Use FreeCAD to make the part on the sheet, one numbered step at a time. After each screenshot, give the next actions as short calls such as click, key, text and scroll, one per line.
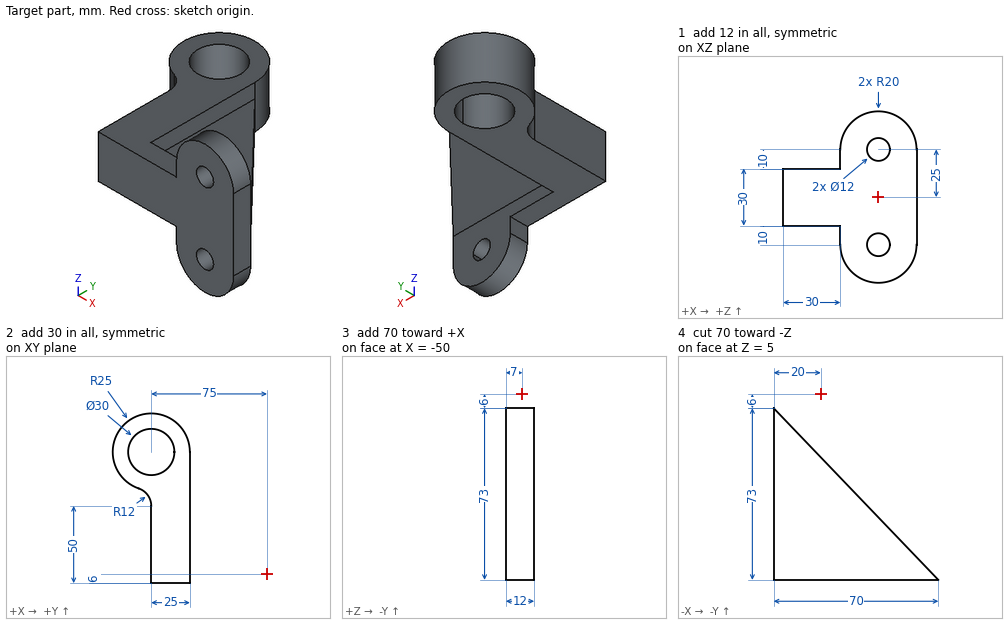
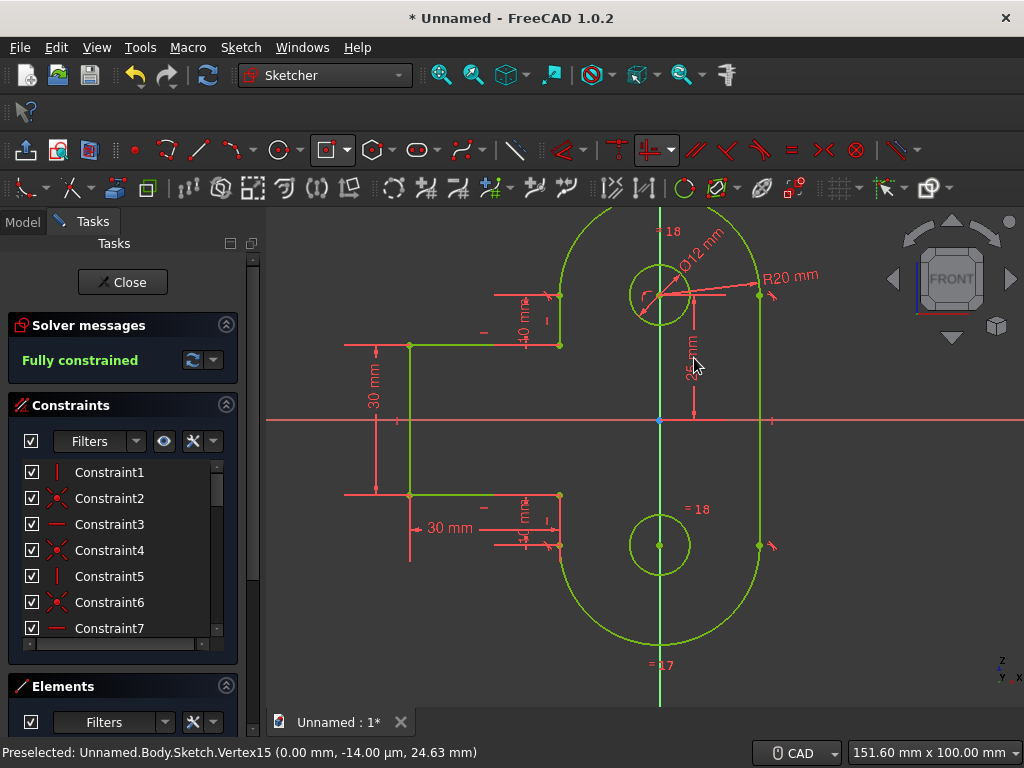
click(123, 282)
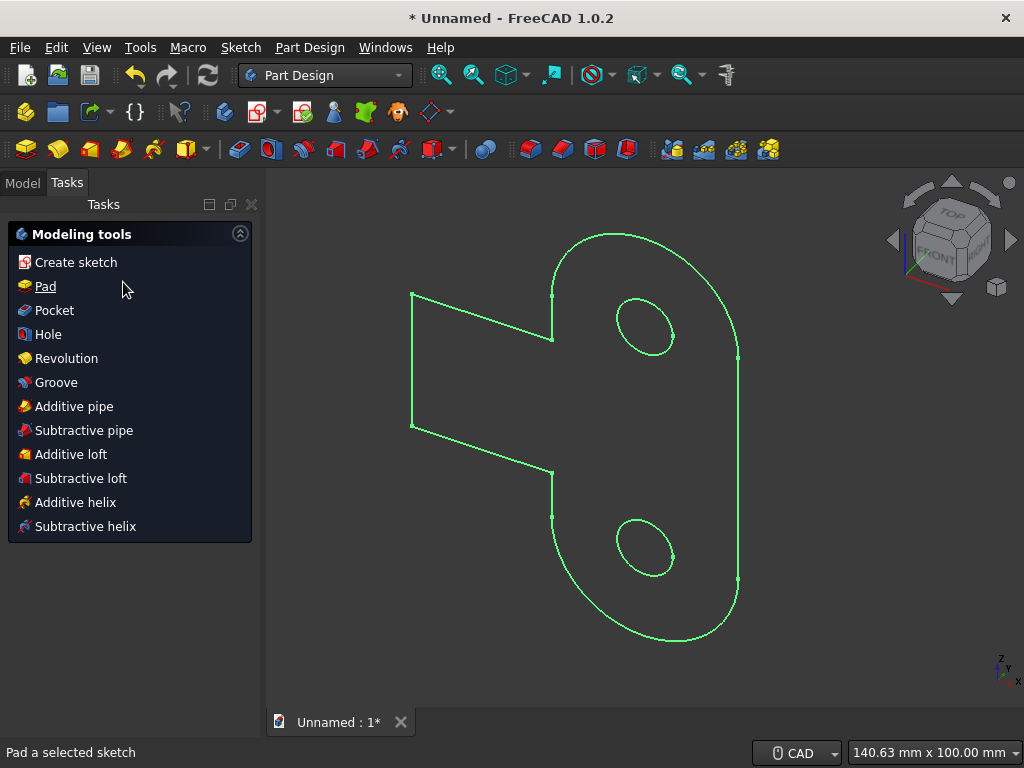
click(26, 150)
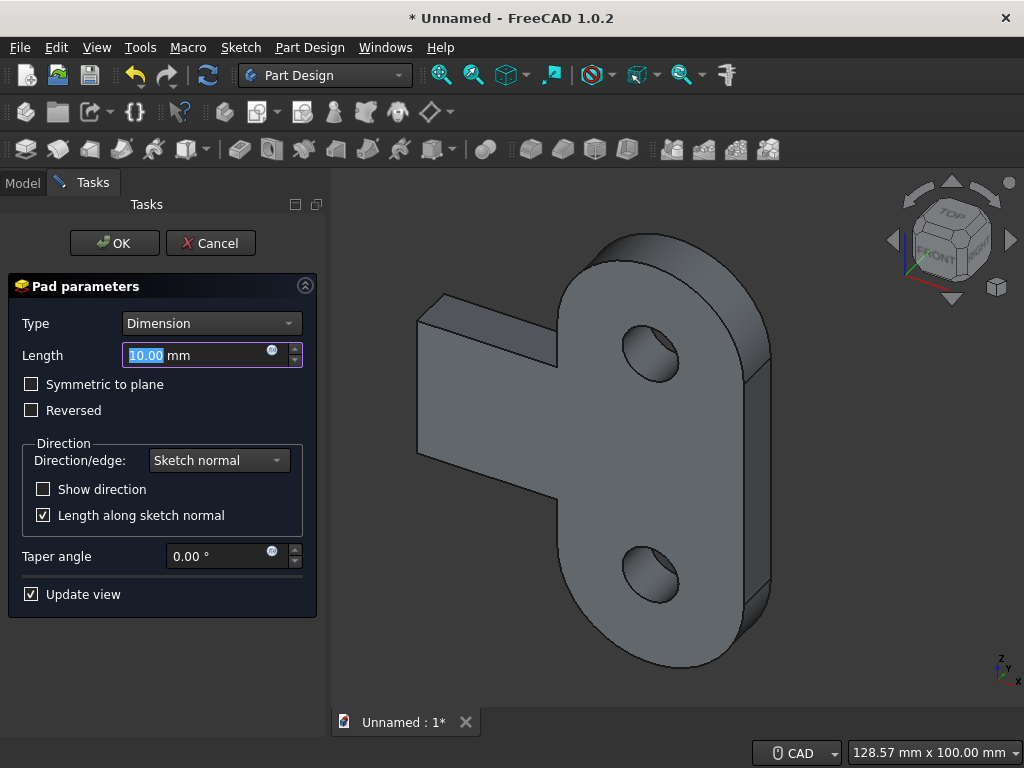
text(12)
key(Tab)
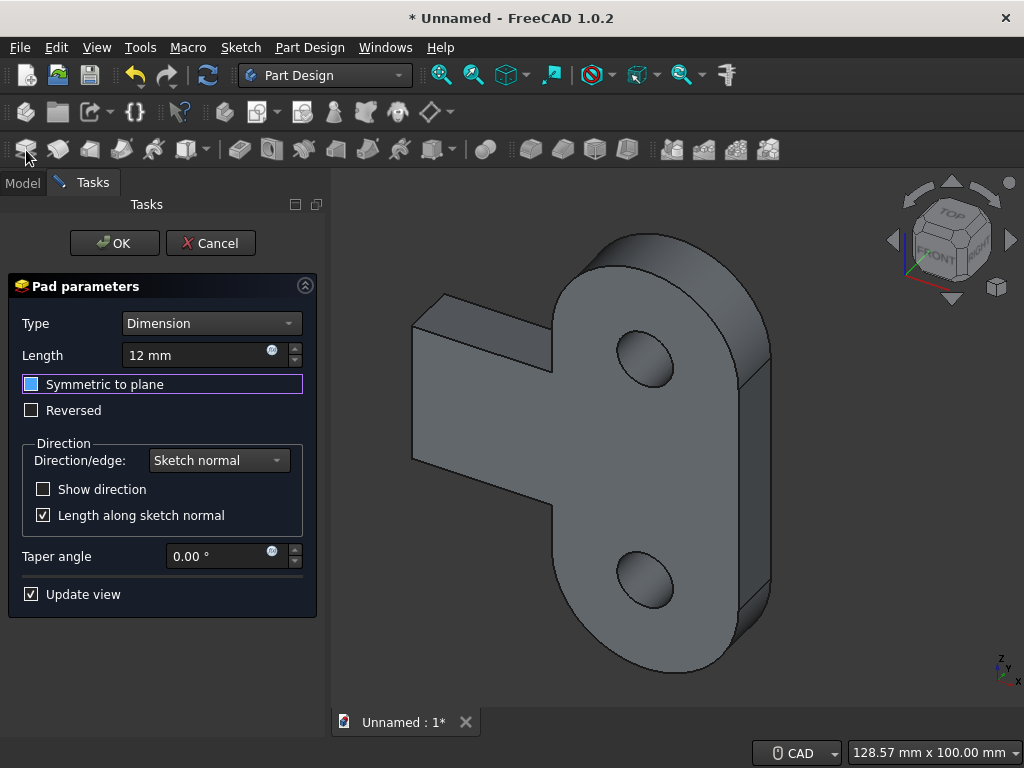
click(30, 384)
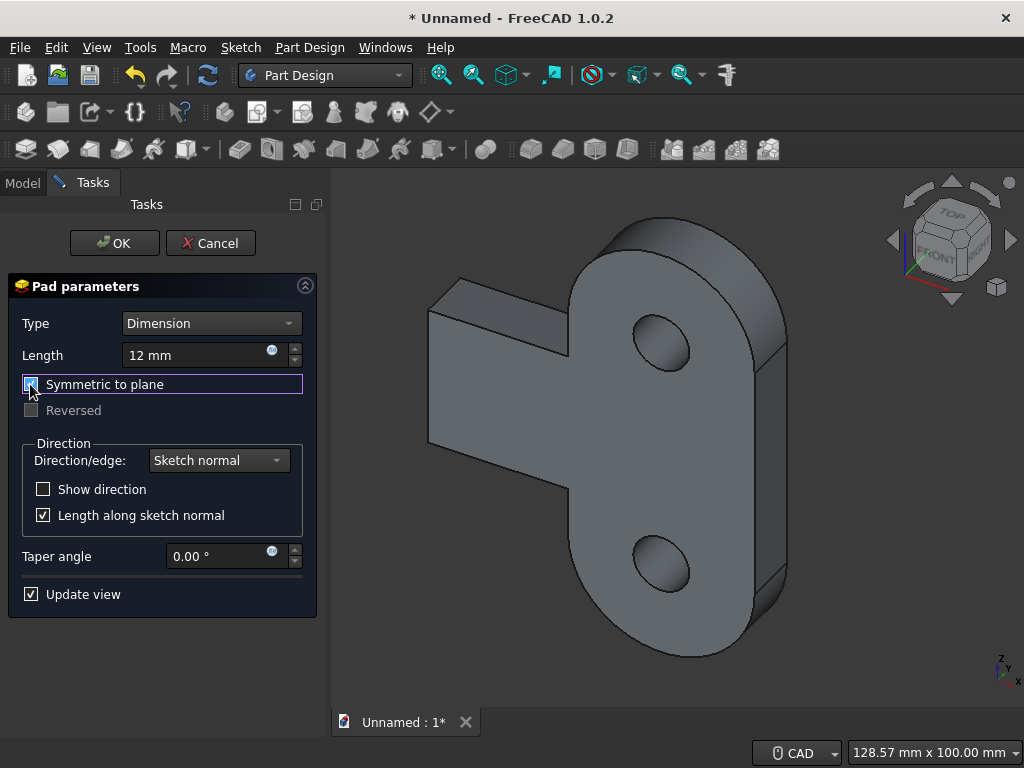
click(115, 243)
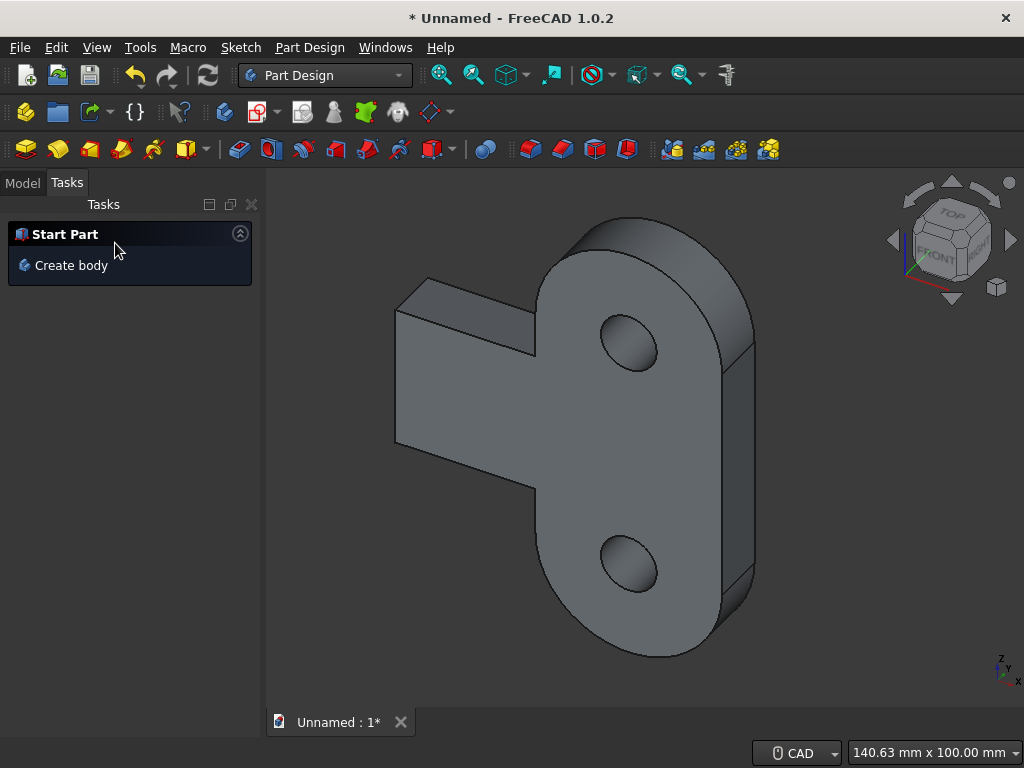
click(442, 76)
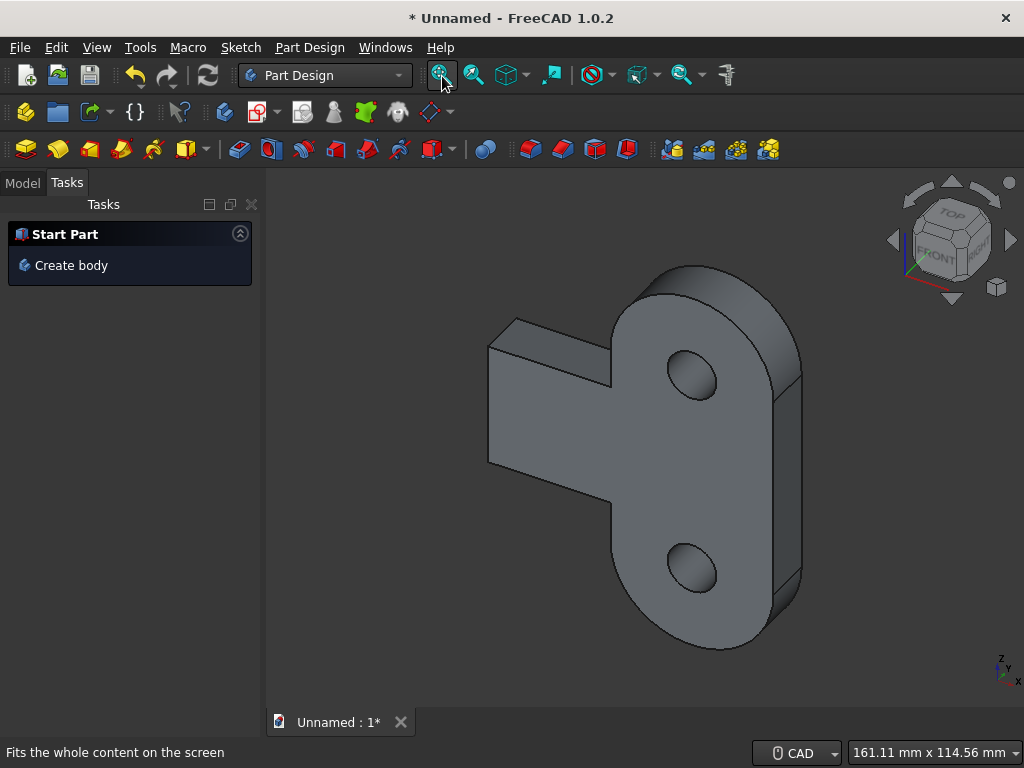
click(258, 112)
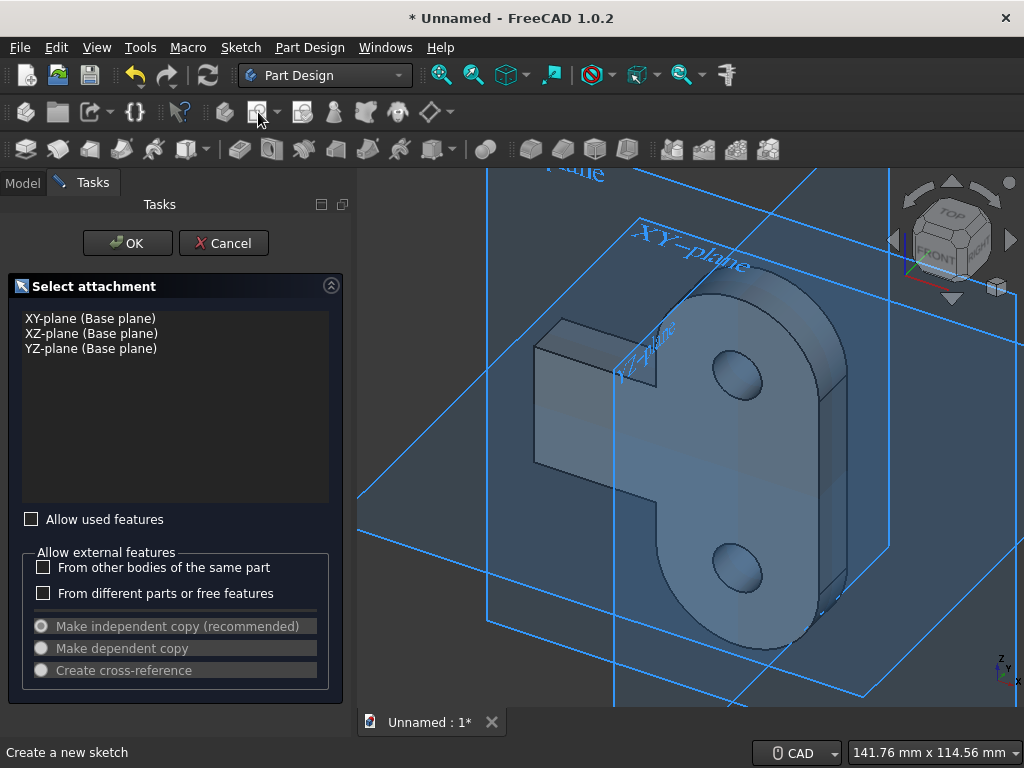
click(82, 318)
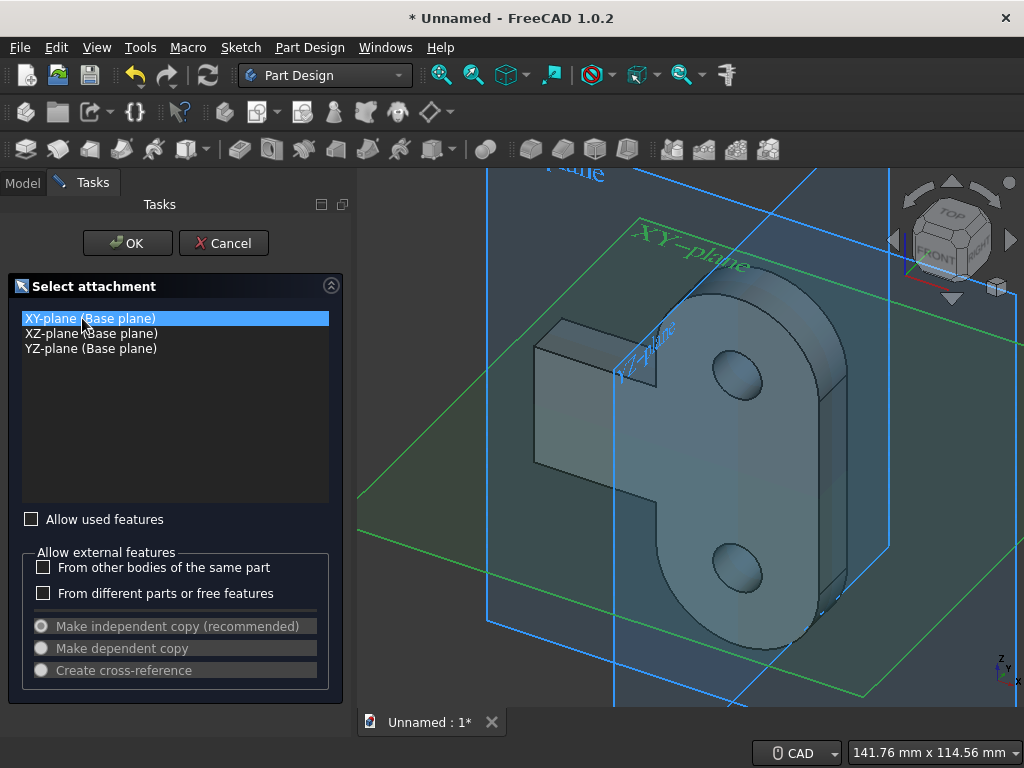
click(128, 243)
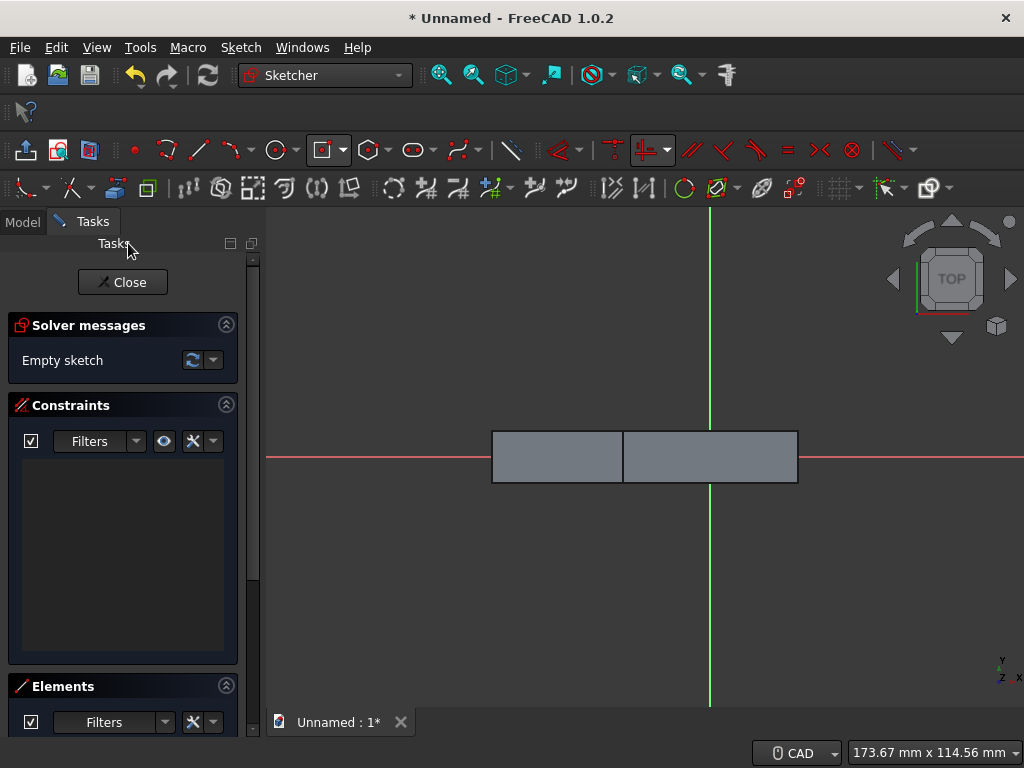
click(90, 150)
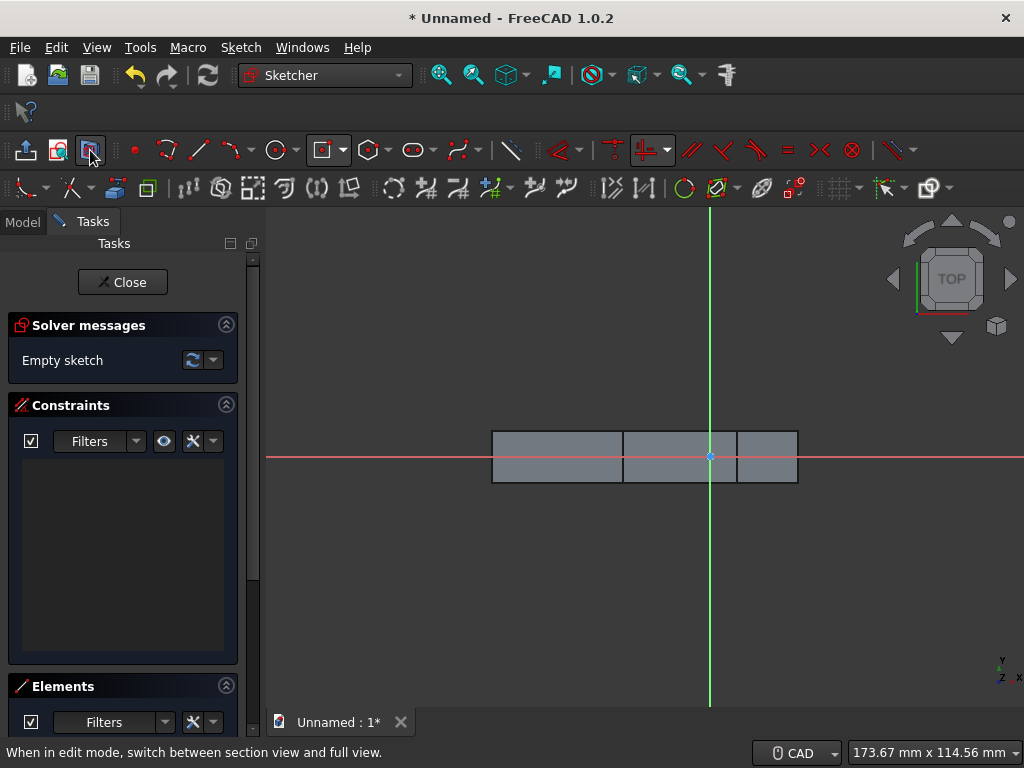
scroll(652, 679, down, 3)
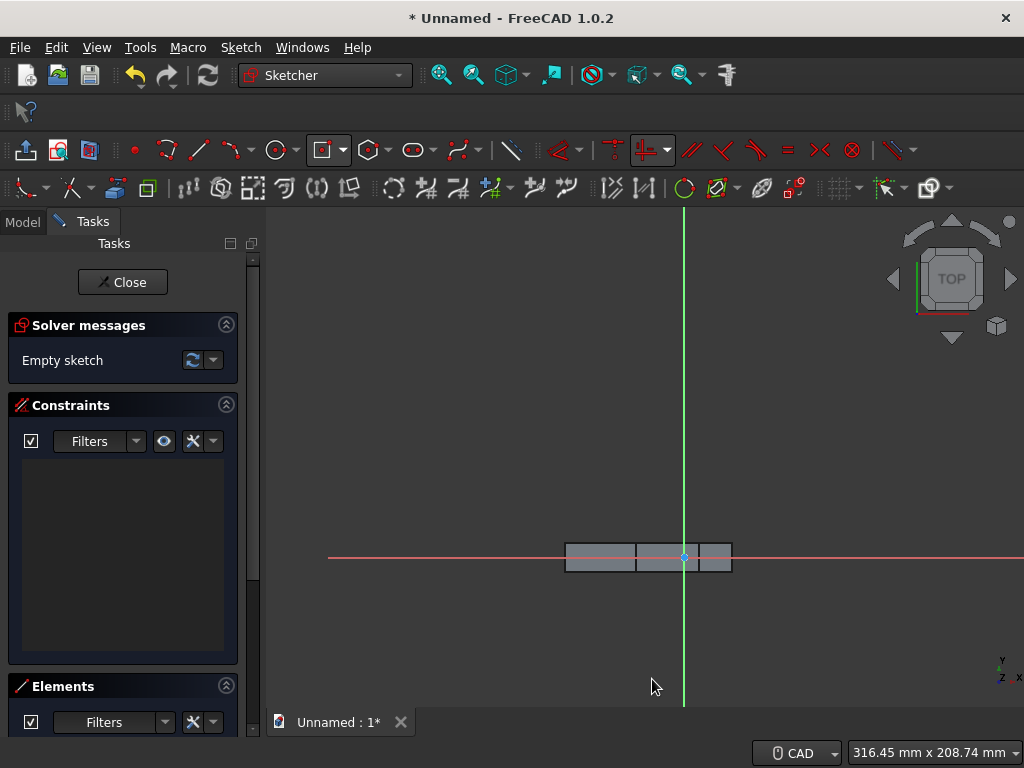
click(168, 150)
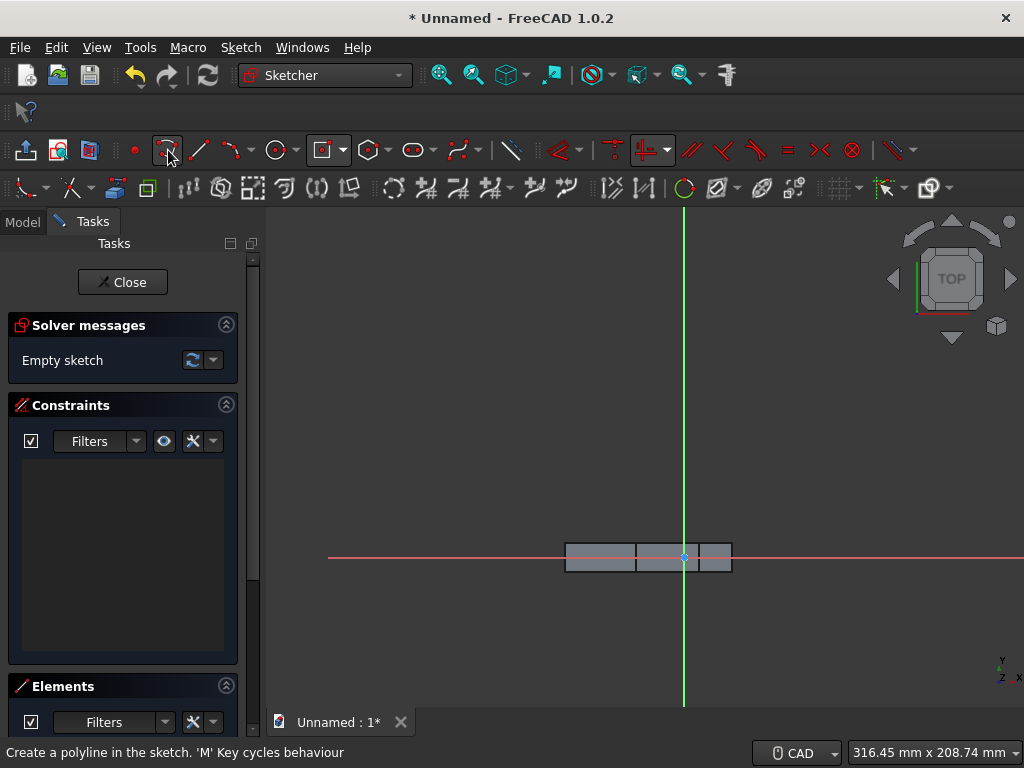
click(505, 452)
click(505, 572)
click(565, 572)
click(565, 368)
right_click(565, 368)